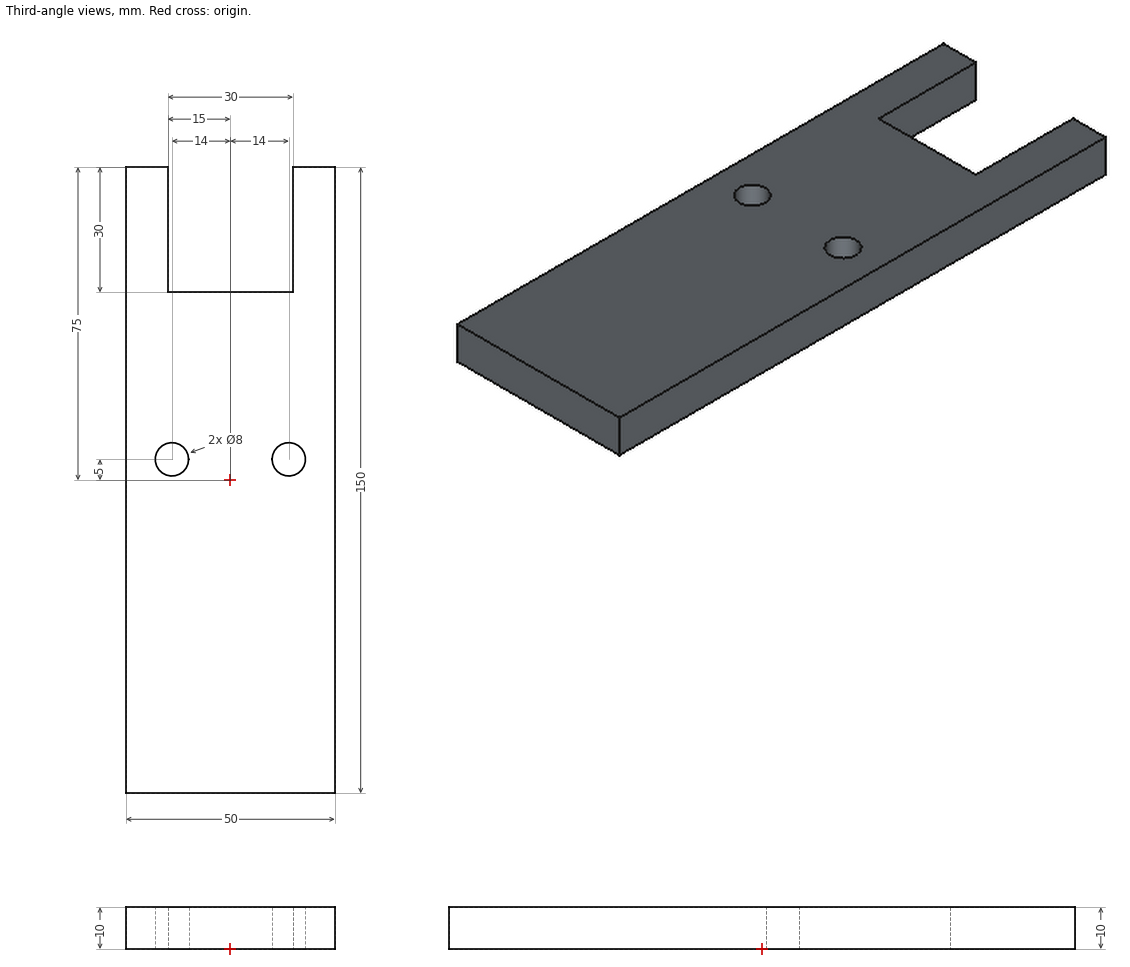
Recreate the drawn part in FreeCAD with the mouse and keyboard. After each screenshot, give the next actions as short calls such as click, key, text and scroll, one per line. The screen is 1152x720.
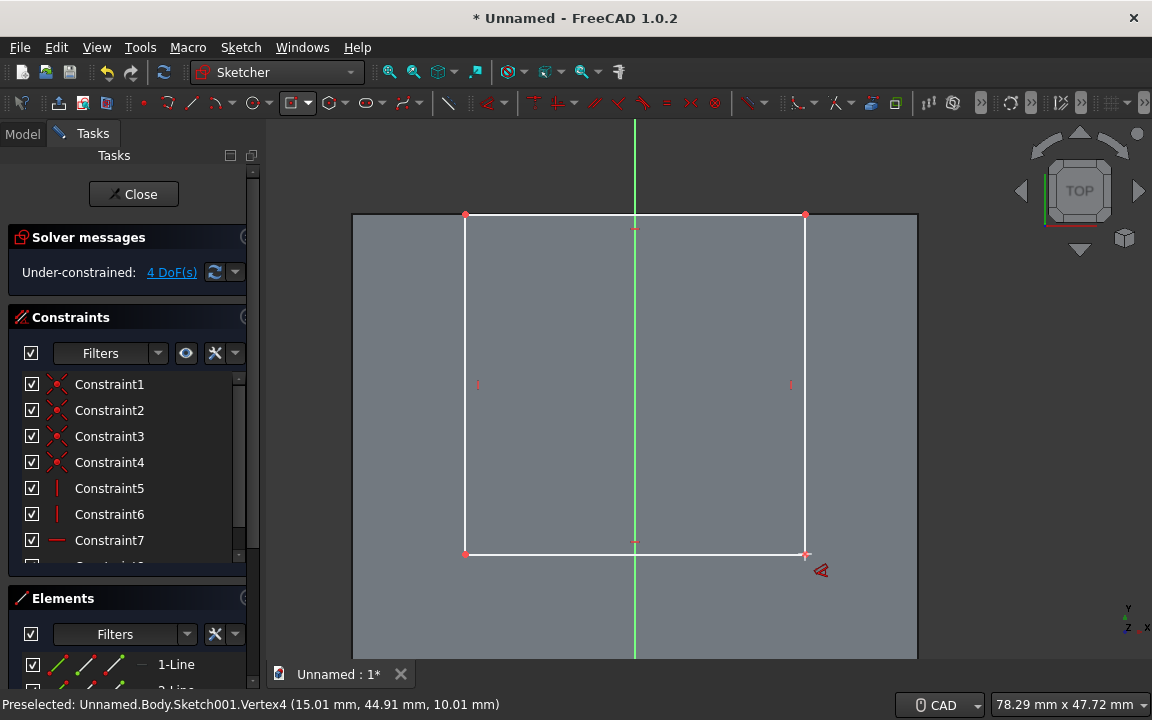
click(465, 317)
click(431, 385)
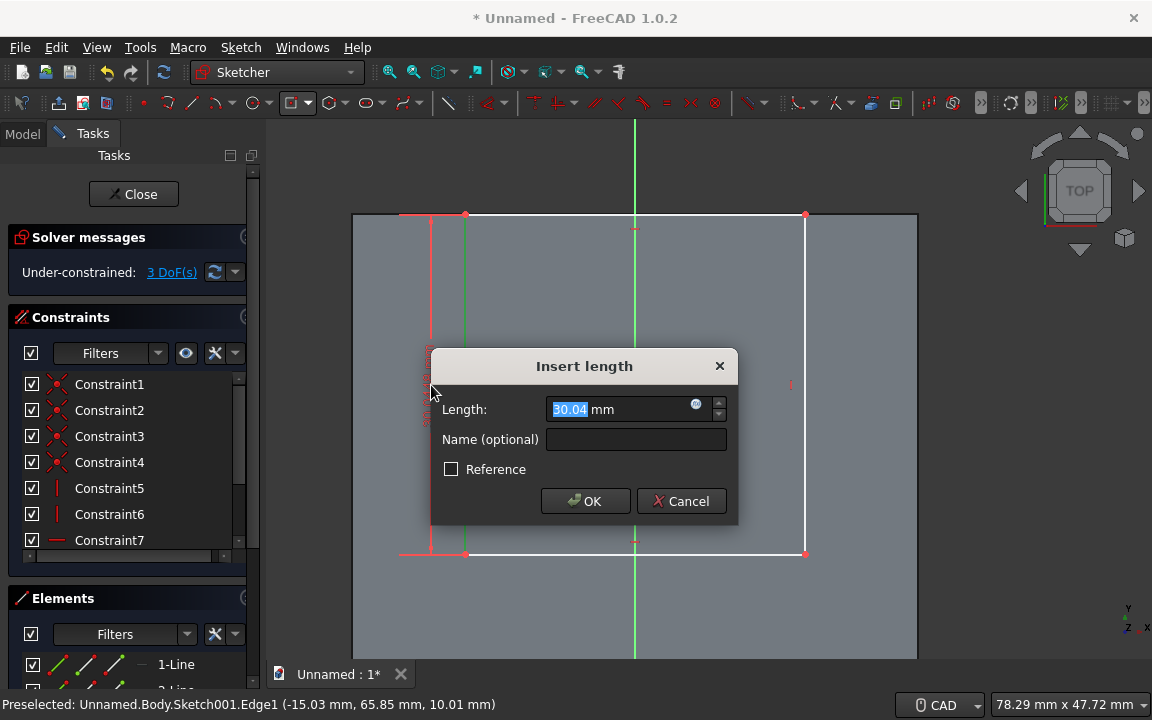
text(30)
key(Return)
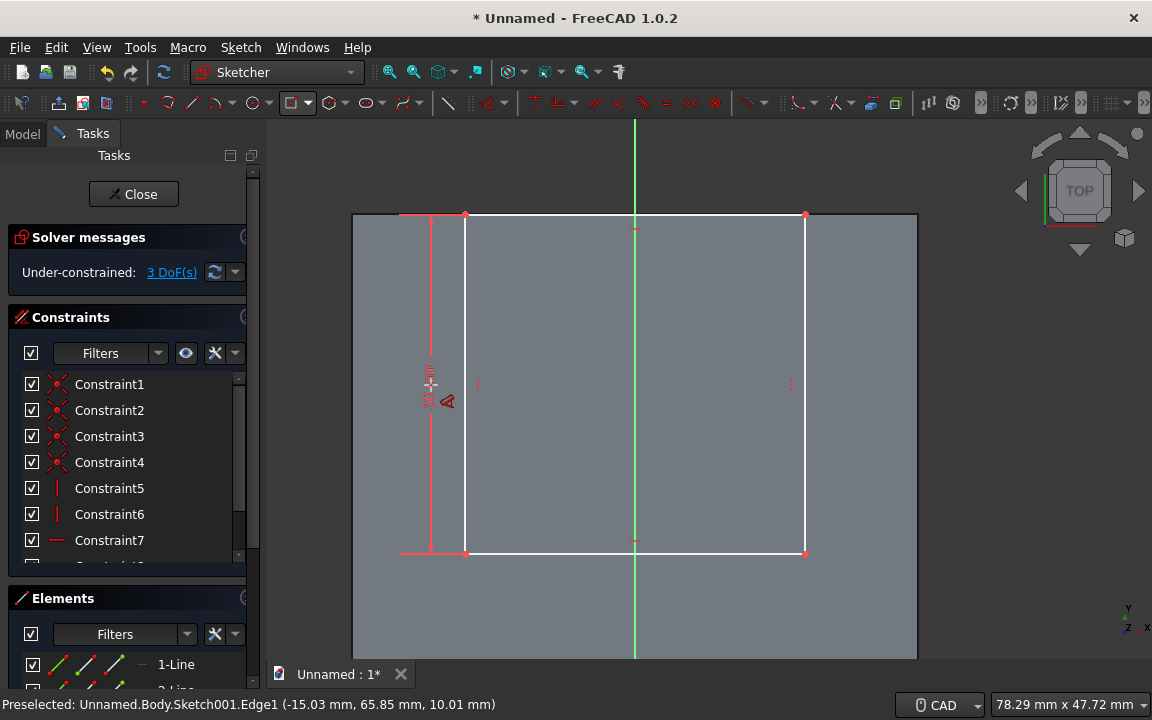
click(567, 554)
click(557, 588)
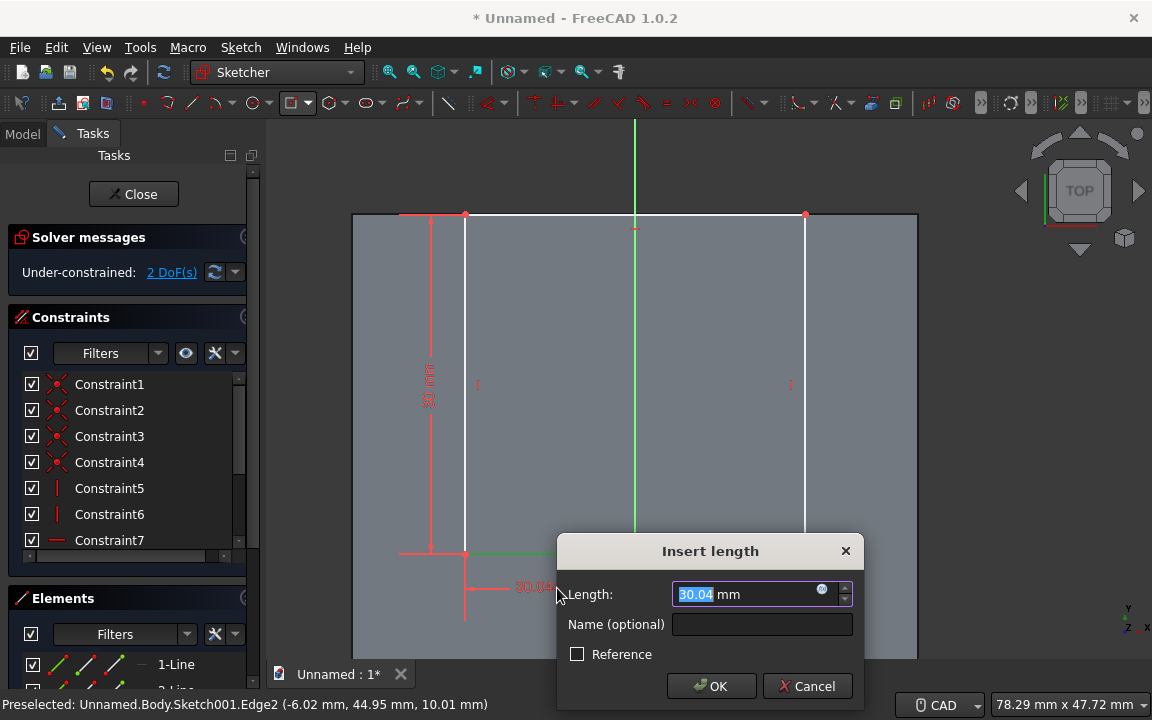
text(30)
key(Return)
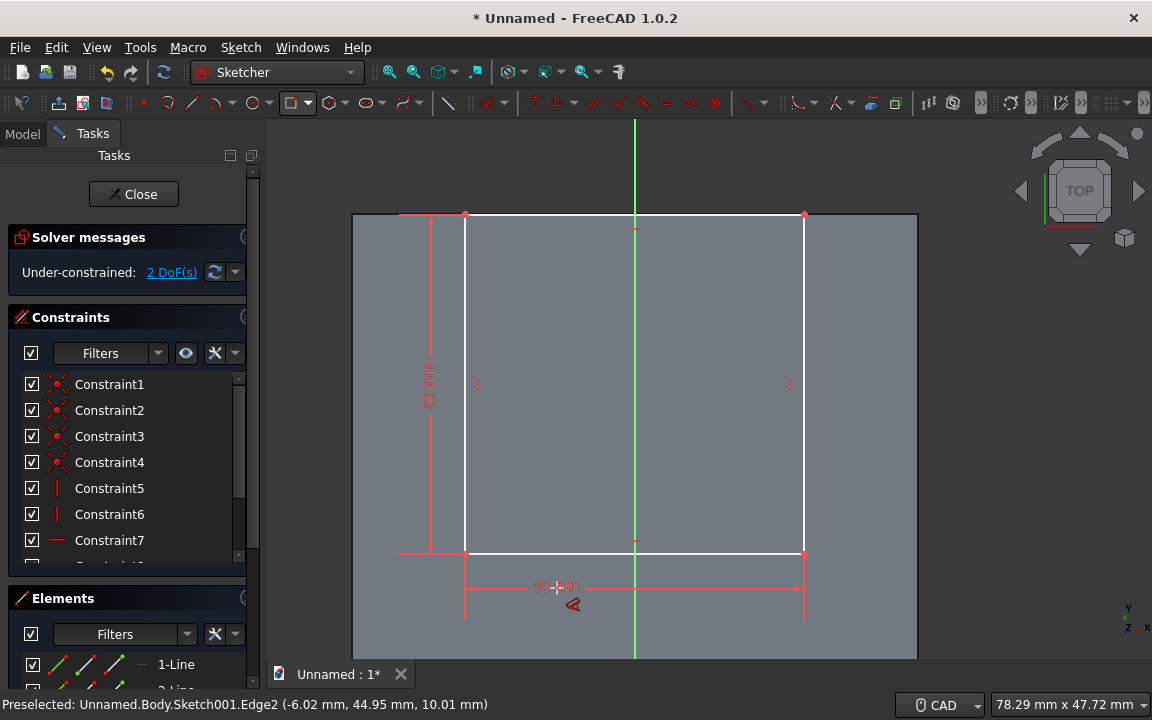
click(465, 215)
click(550, 181)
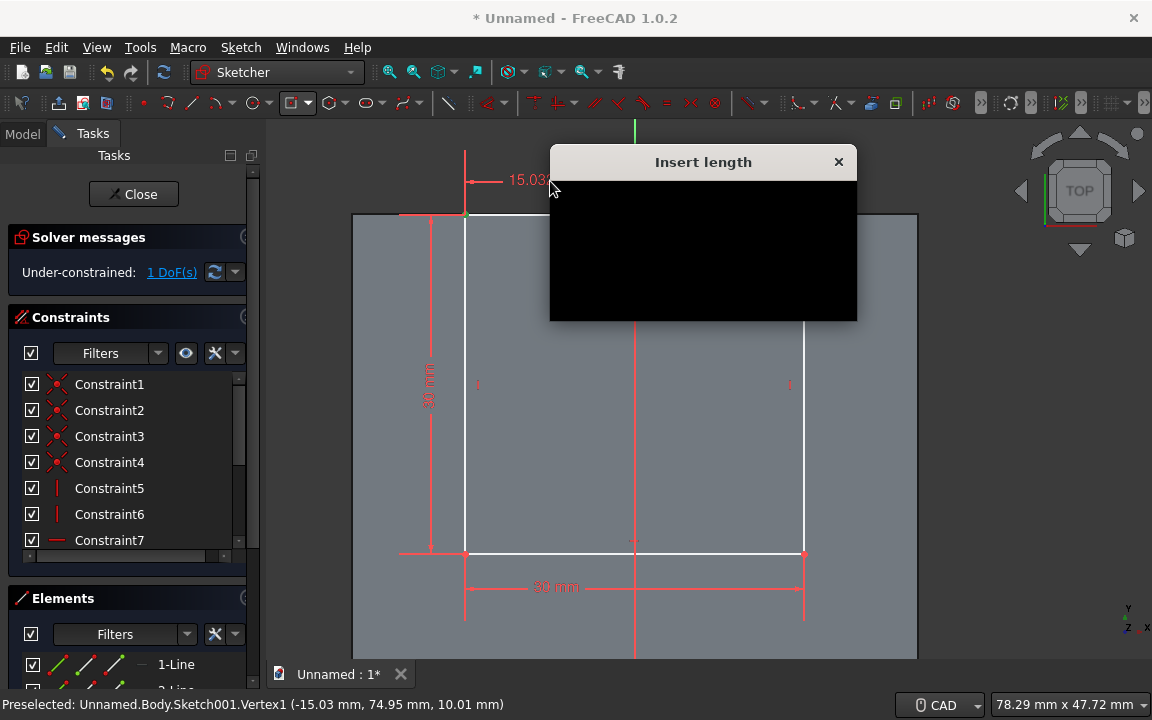
text(15)
key(Return)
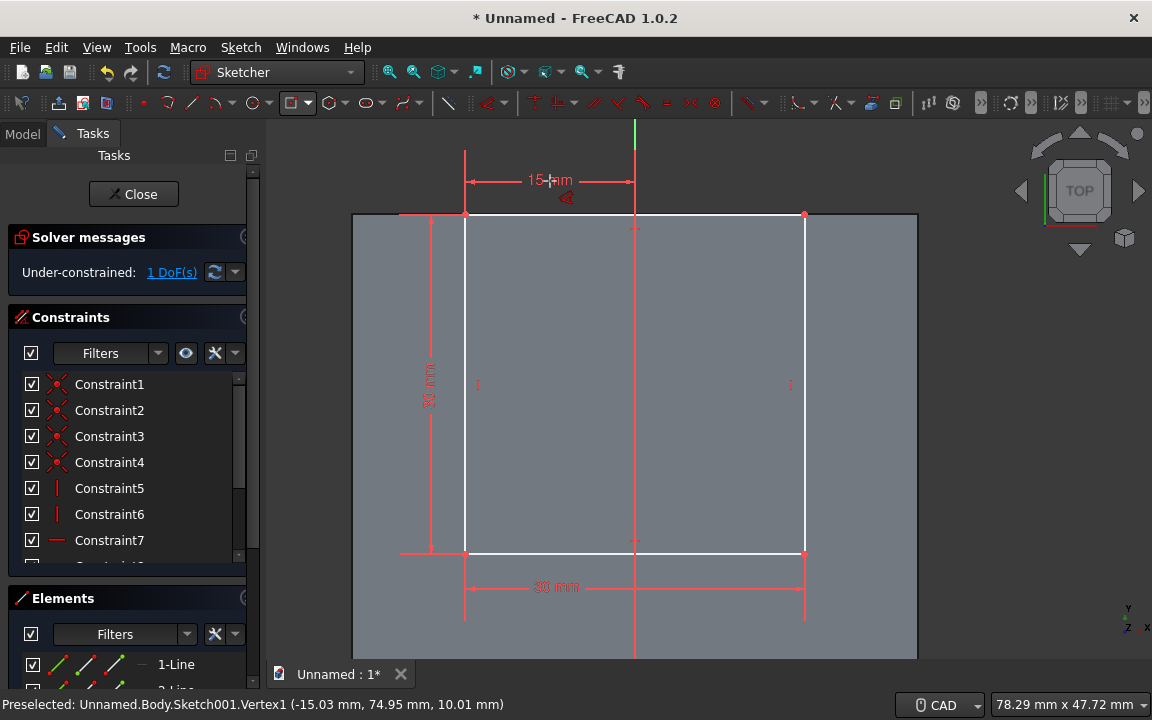
click(465, 215)
click(431, 423)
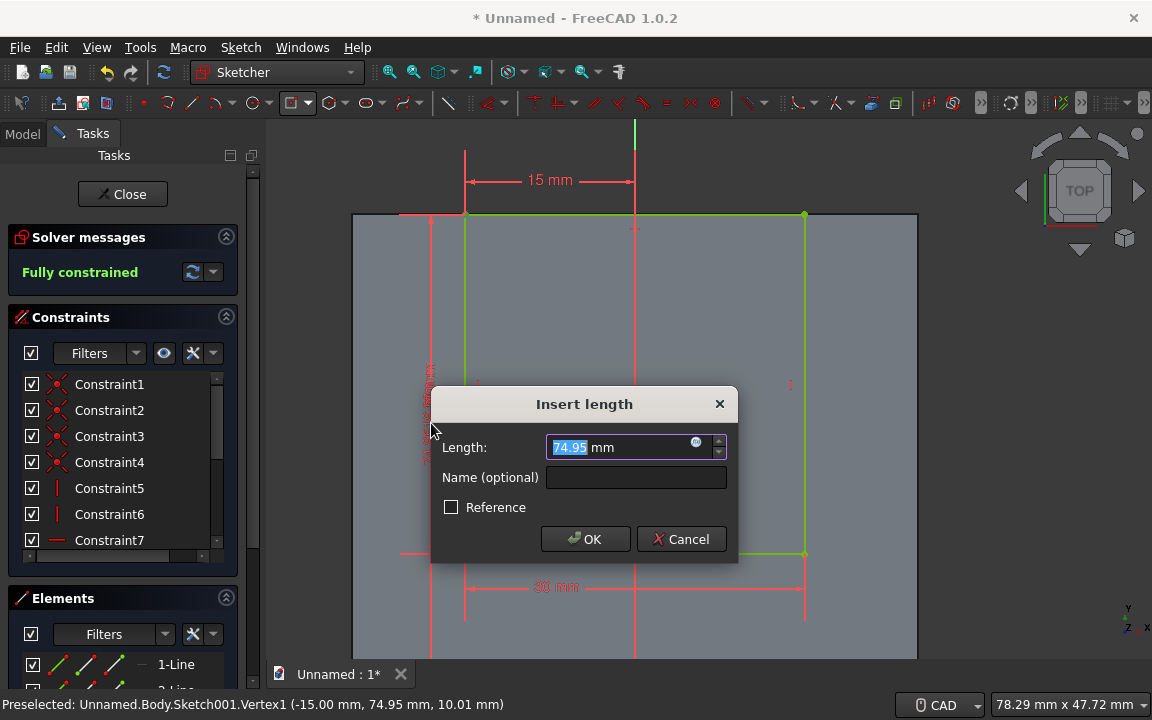
text(75)
key(Return)
key(Escape)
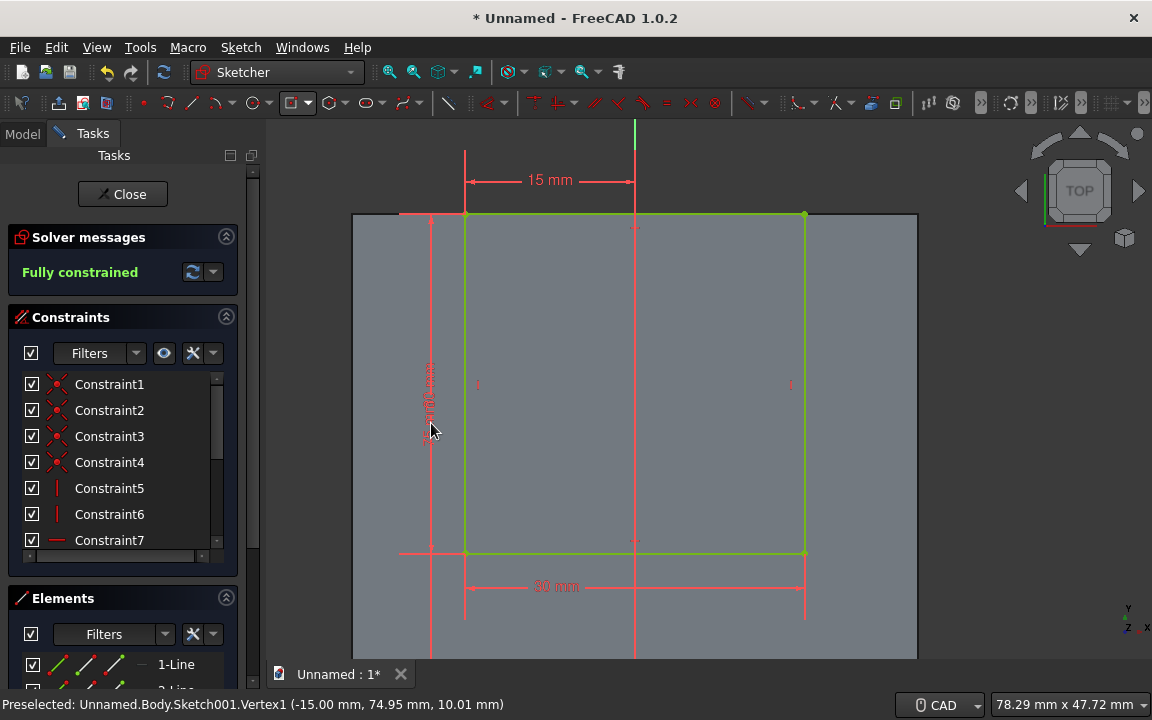
click(123, 194)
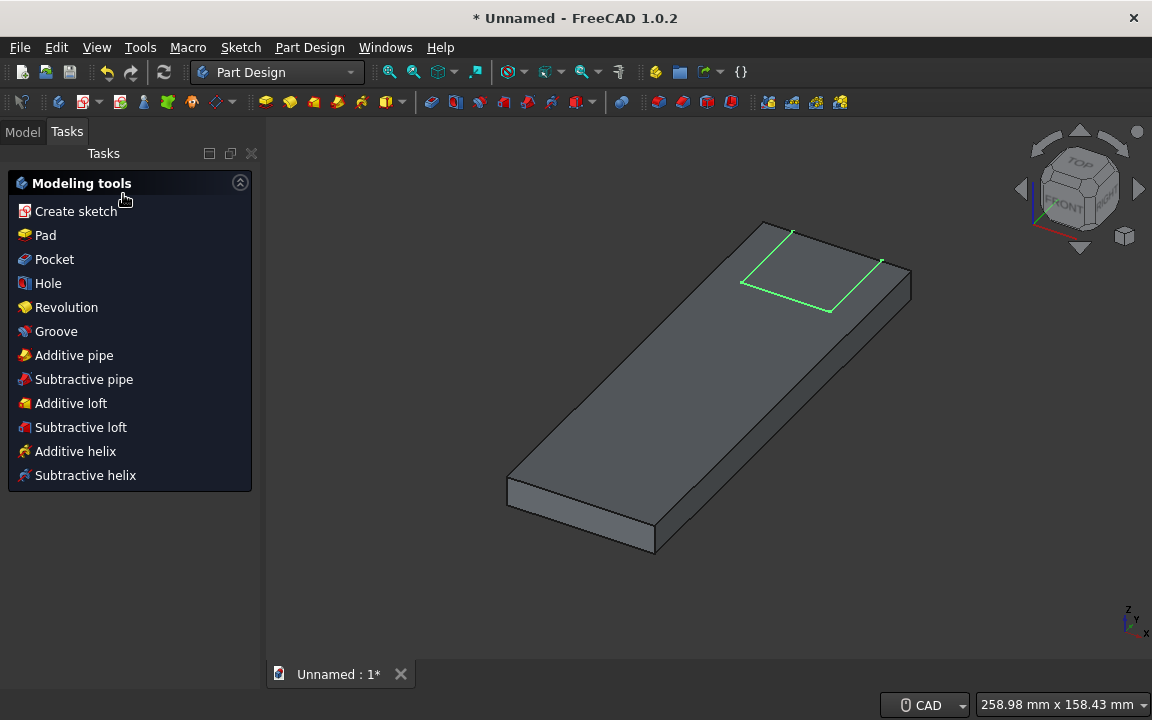
click(432, 102)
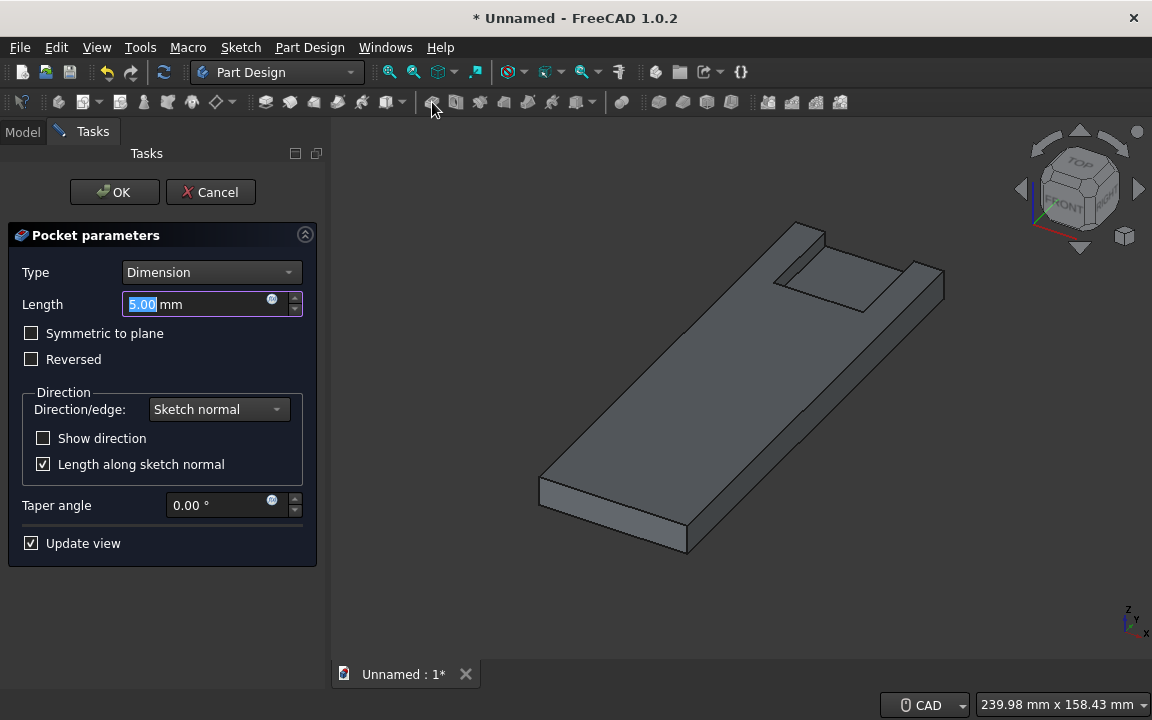
text(10)
key(Tab)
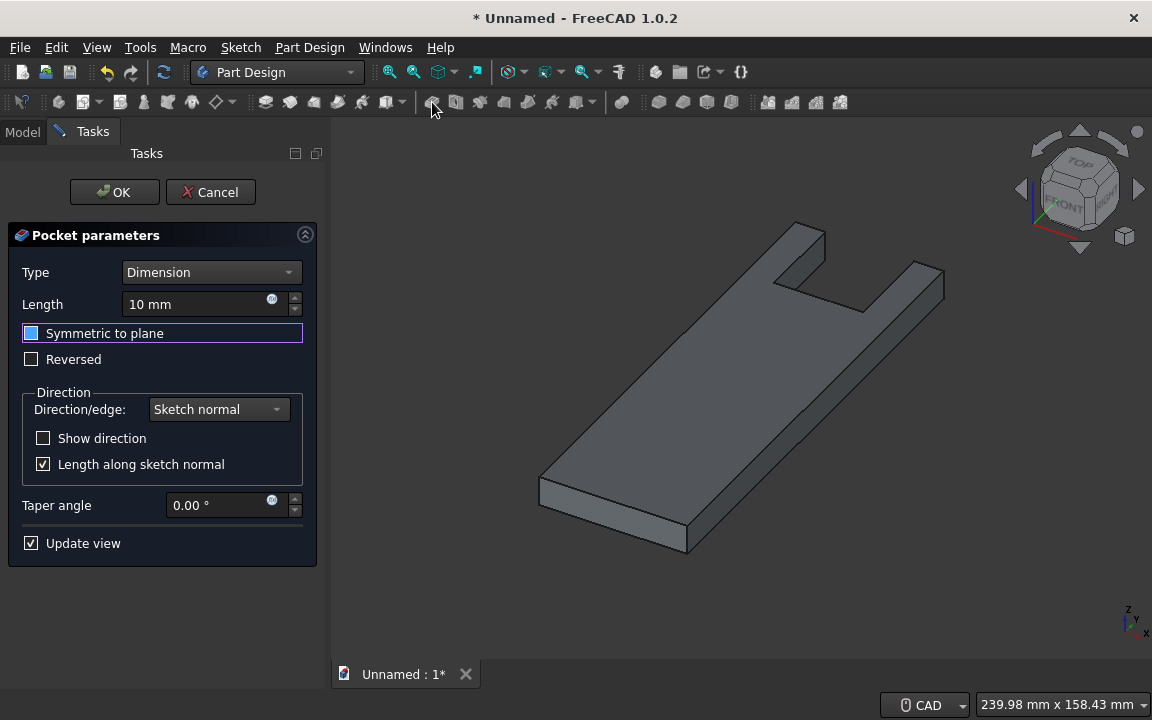
click(115, 192)